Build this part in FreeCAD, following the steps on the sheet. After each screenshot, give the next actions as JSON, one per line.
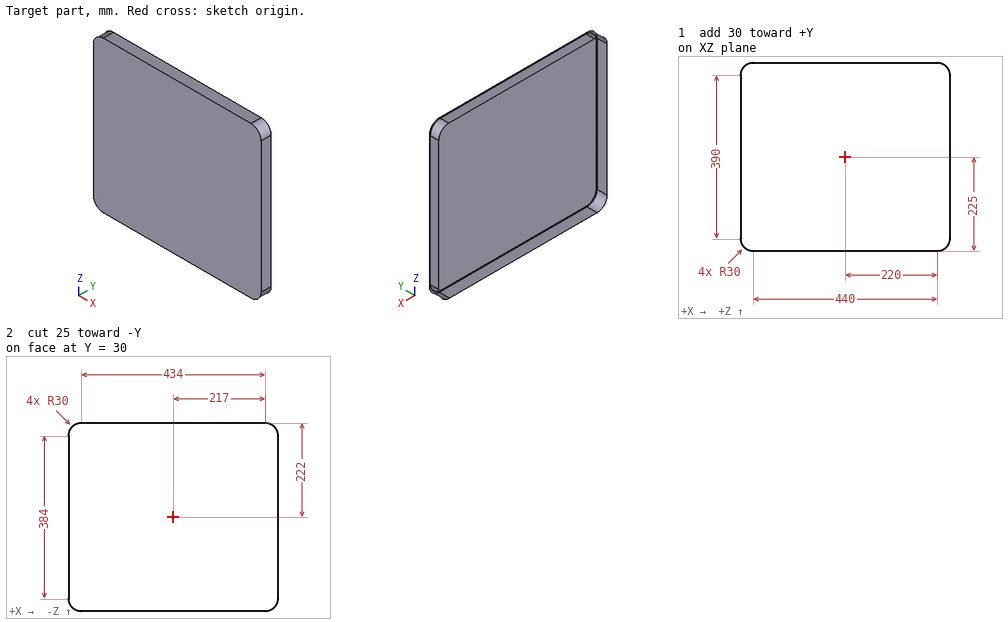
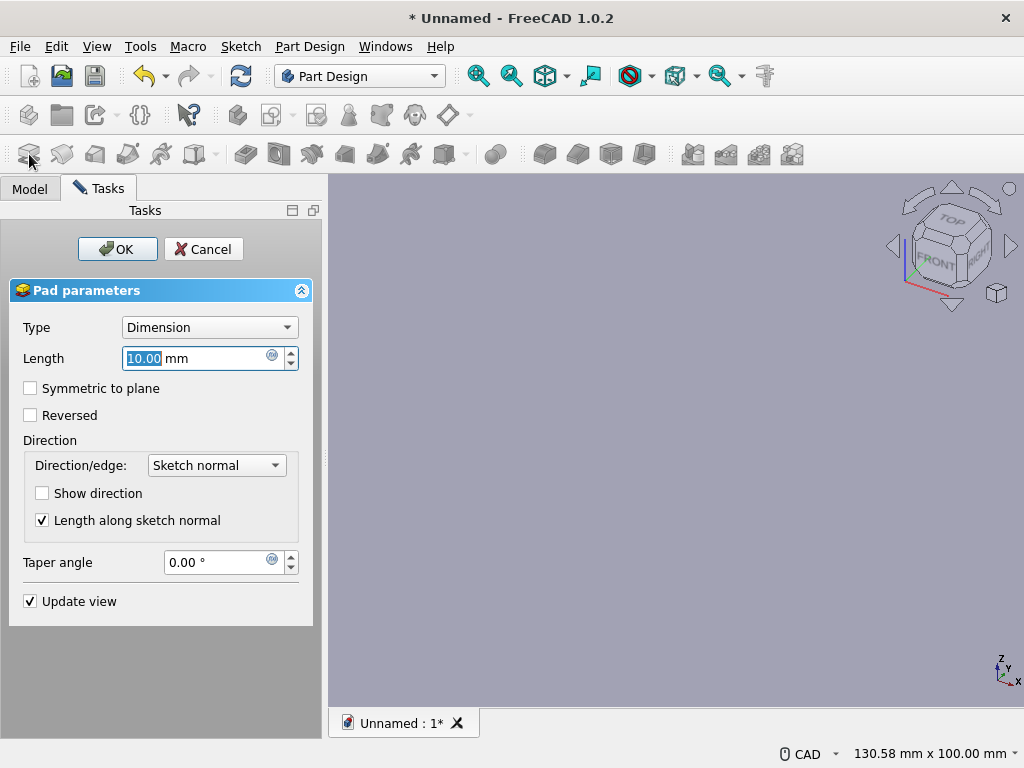
{"action": "type", "text": "30"}
{"action": "key", "text": "Tab"}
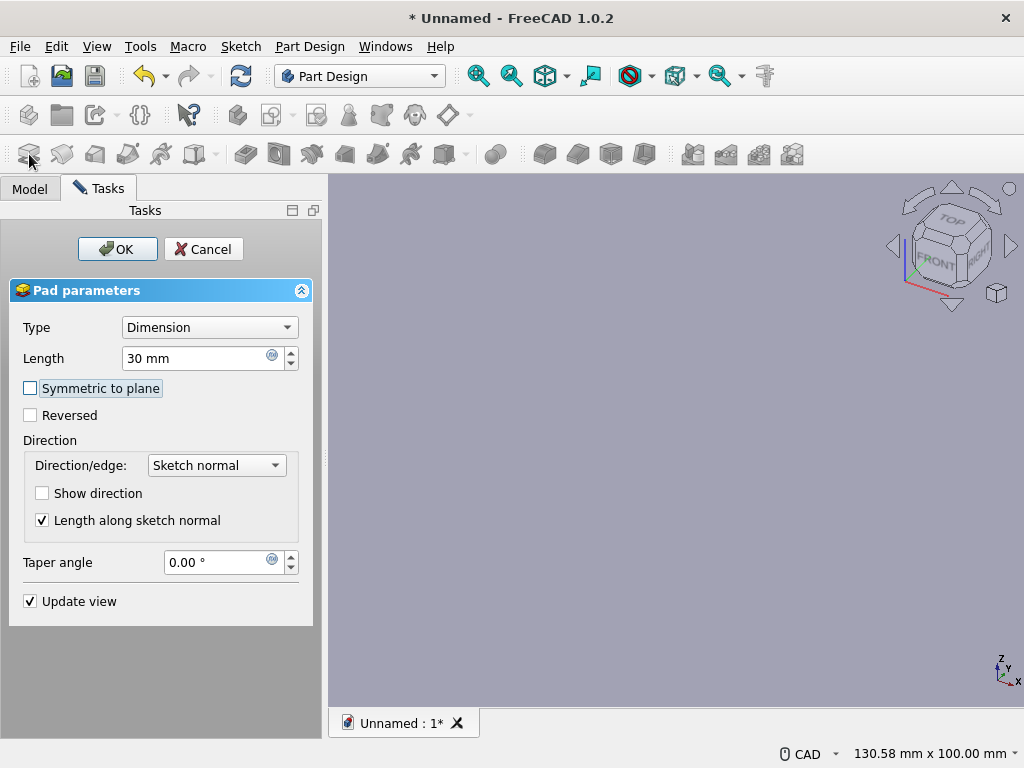
{"action": "left_click", "coordinate": [31, 415]}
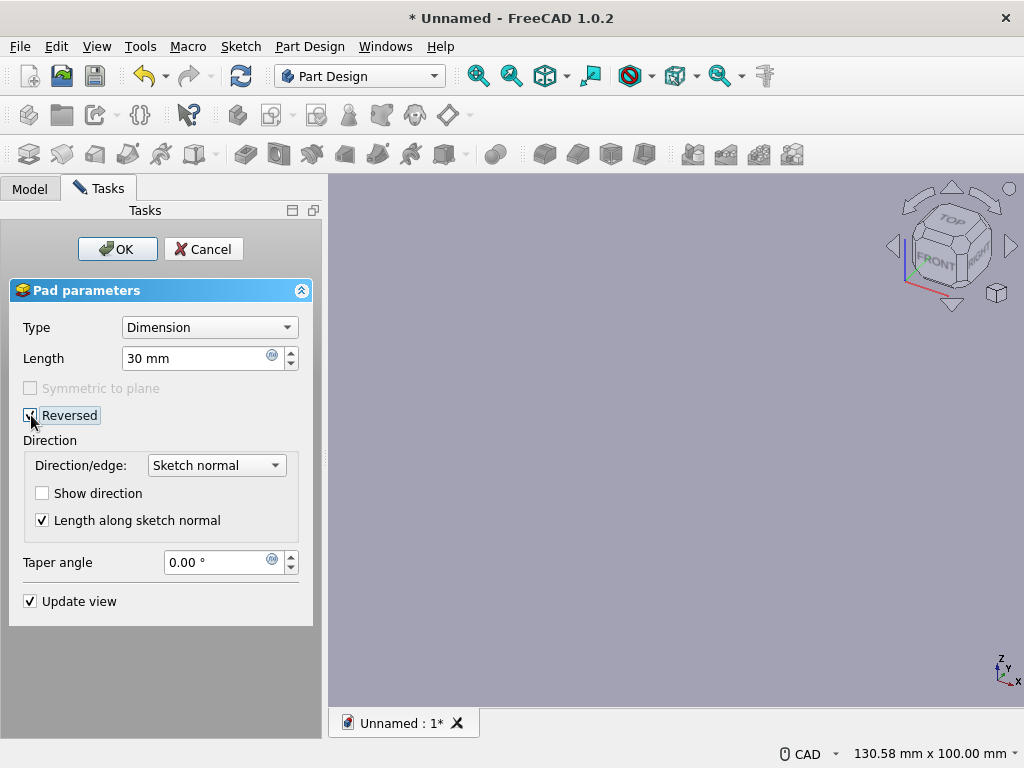
{"action": "left_click", "coordinate": [118, 249]}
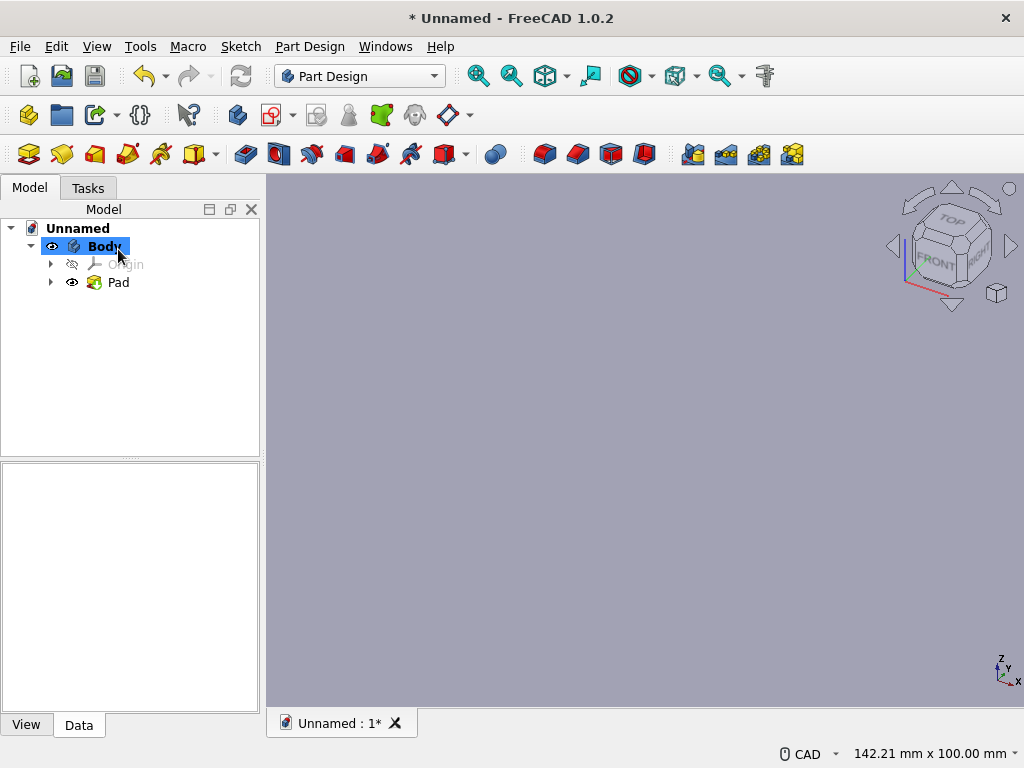
{"action": "left_click", "coordinate": [479, 76]}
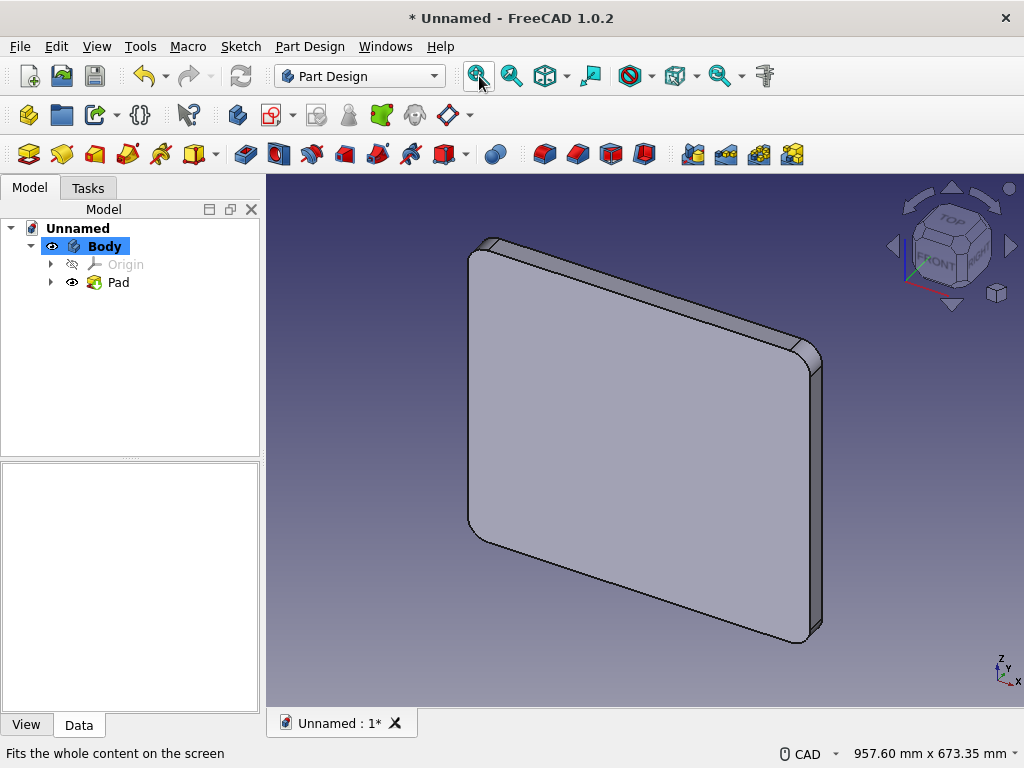
{"action": "key", "text": "4"}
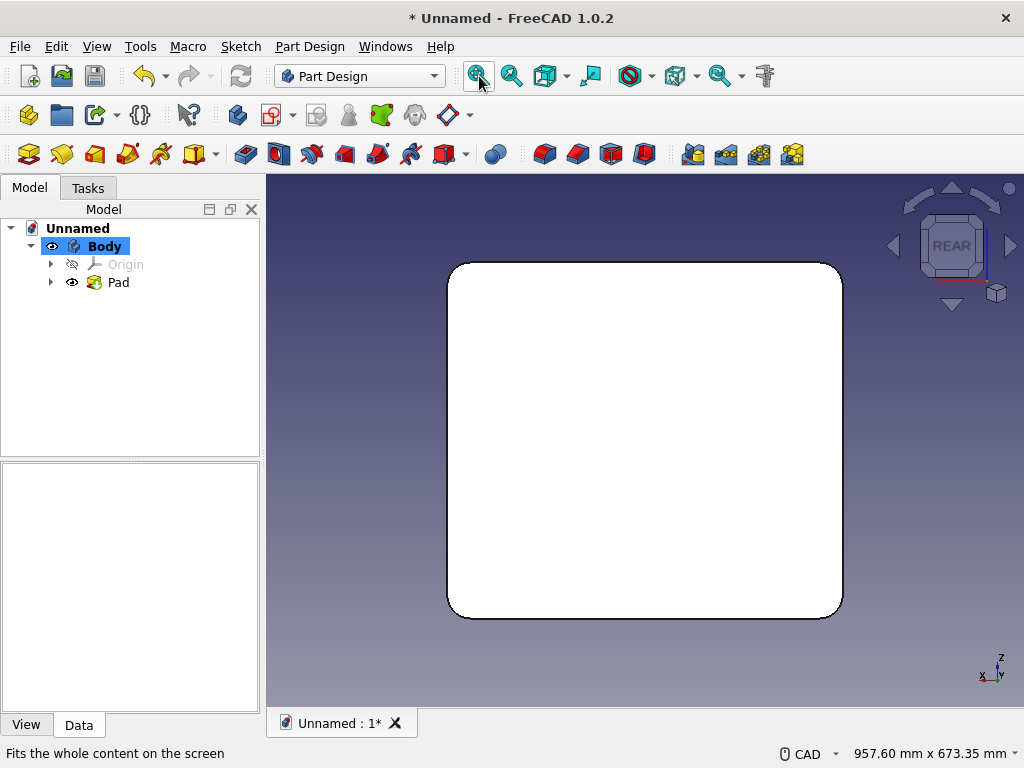
{"action": "left_click", "coordinate": [645, 439]}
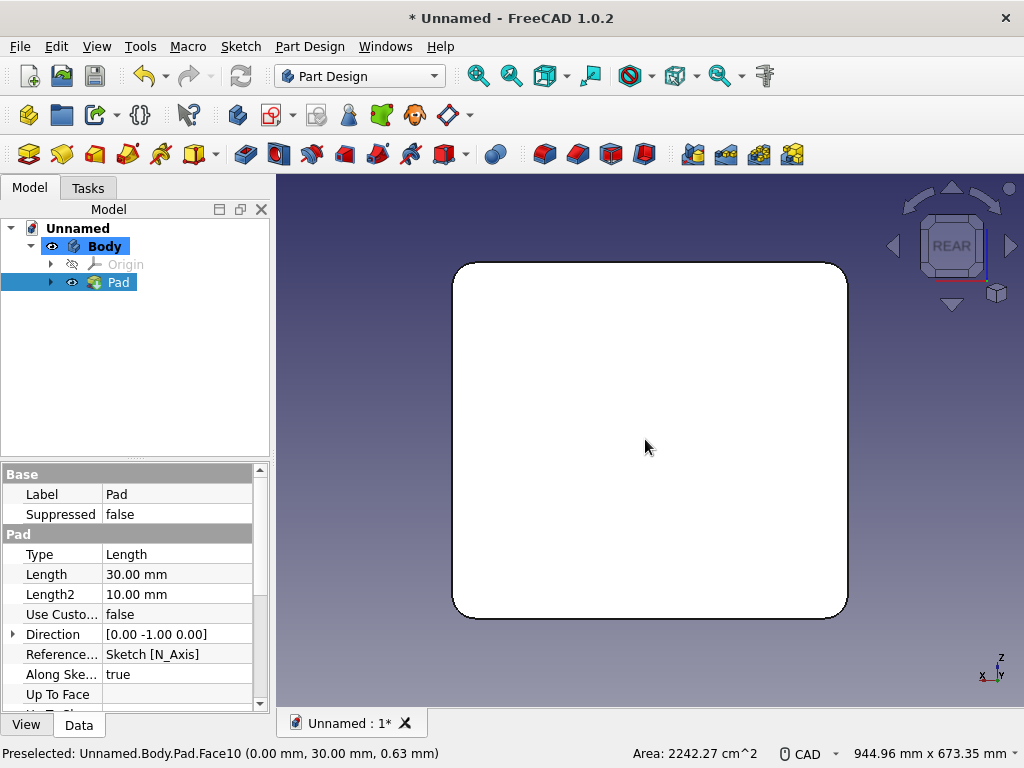
{"action": "left_click", "coordinate": [270, 116]}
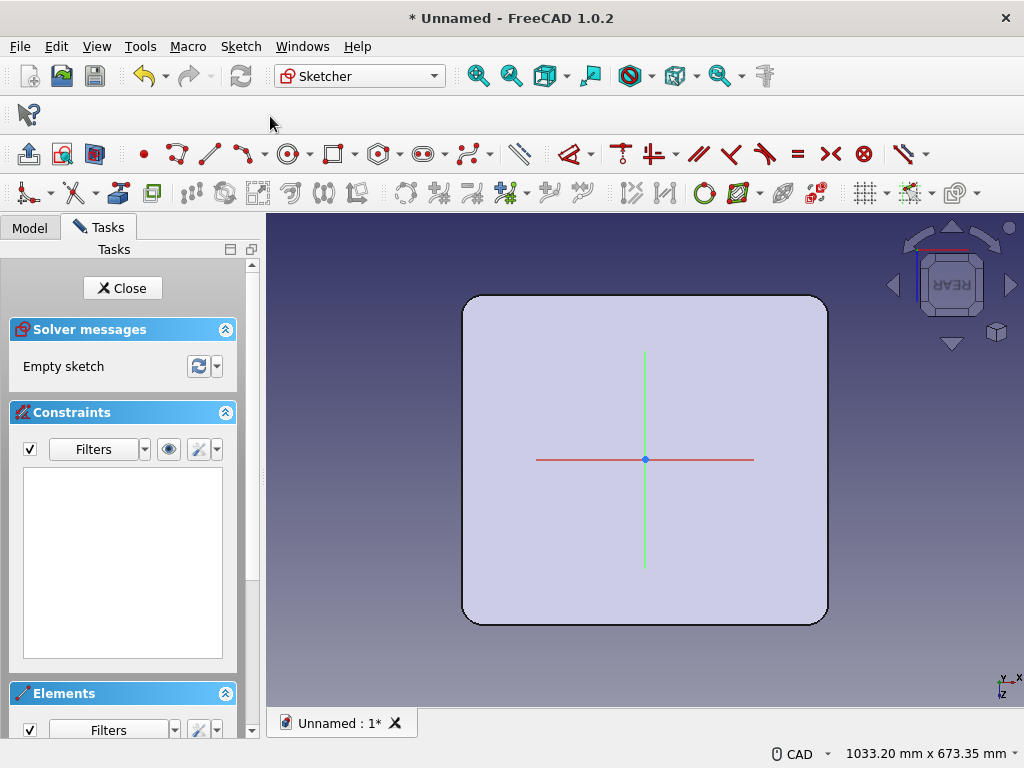
{"action": "left_click", "coordinate": [210, 154]}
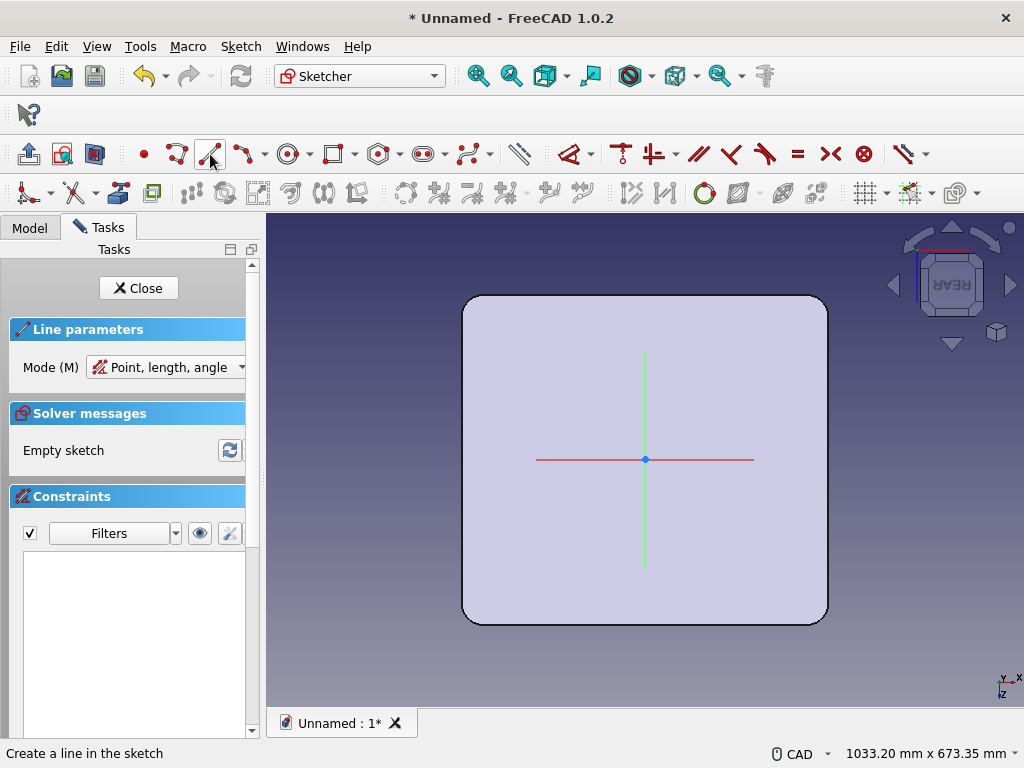
{"action": "left_click", "coordinate": [804, 297]}
{"action": "left_click", "coordinate": [486, 297]}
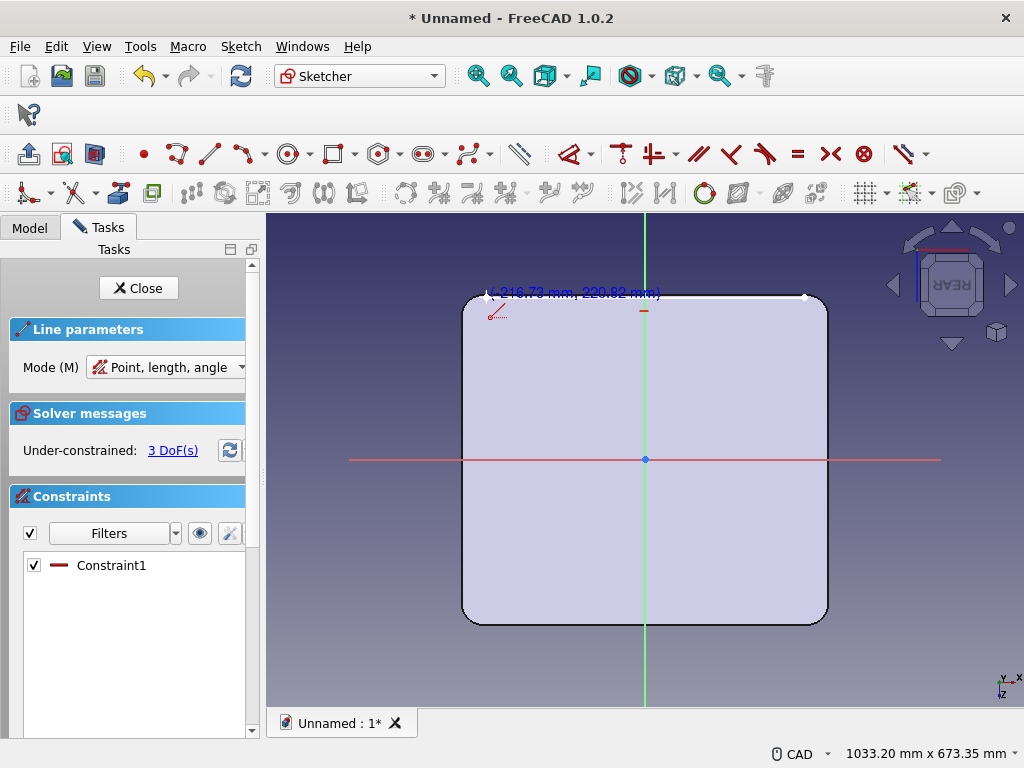
{"action": "left_click", "coordinate": [464, 319]}
{"action": "left_click", "coordinate": [464, 601]}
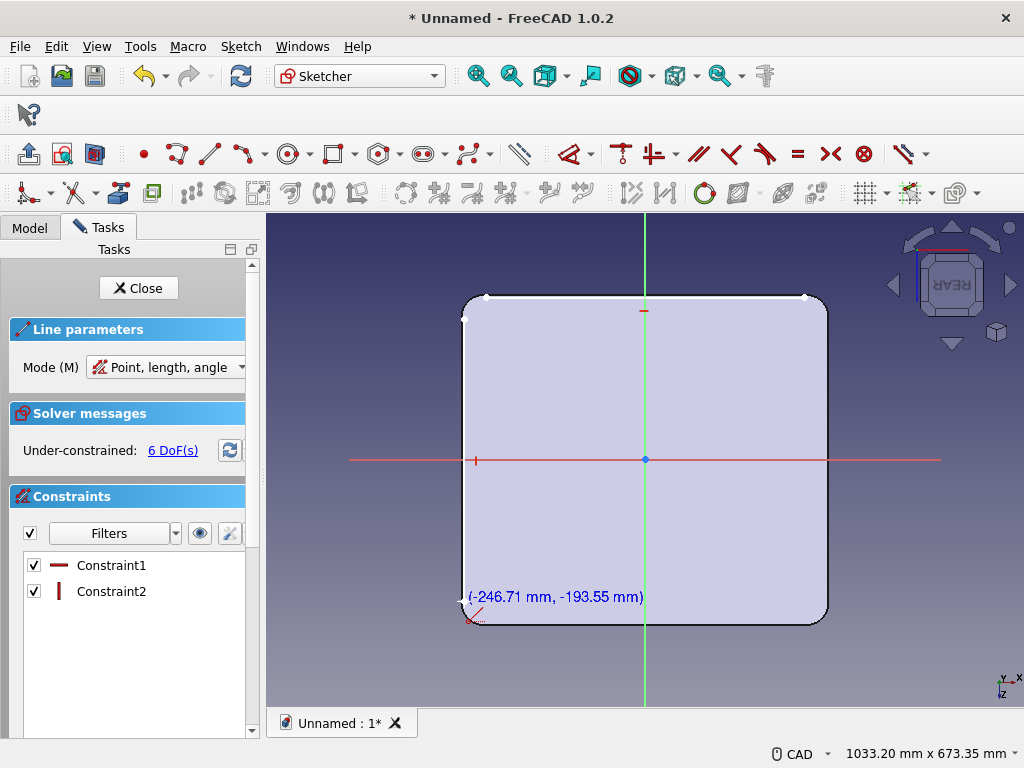
{"action": "left_click", "coordinate": [486, 623]}
{"action": "left_click", "coordinate": [804, 623]}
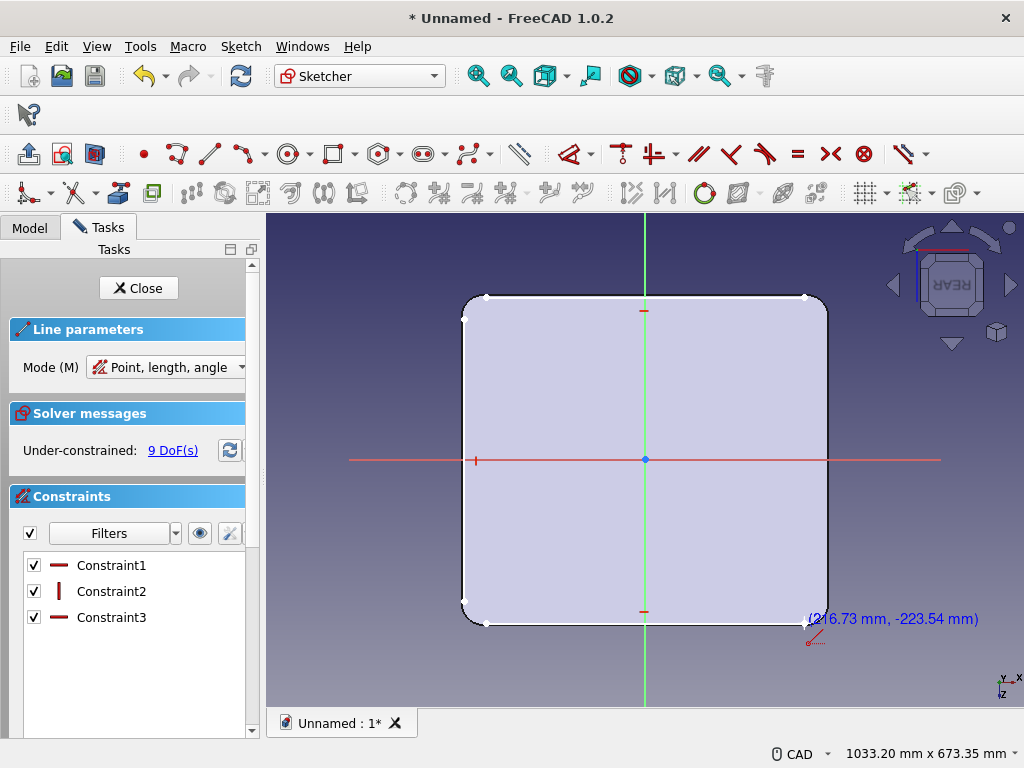
{"action": "left_click", "coordinate": [826, 601]}
{"action": "left_click", "coordinate": [826, 319]}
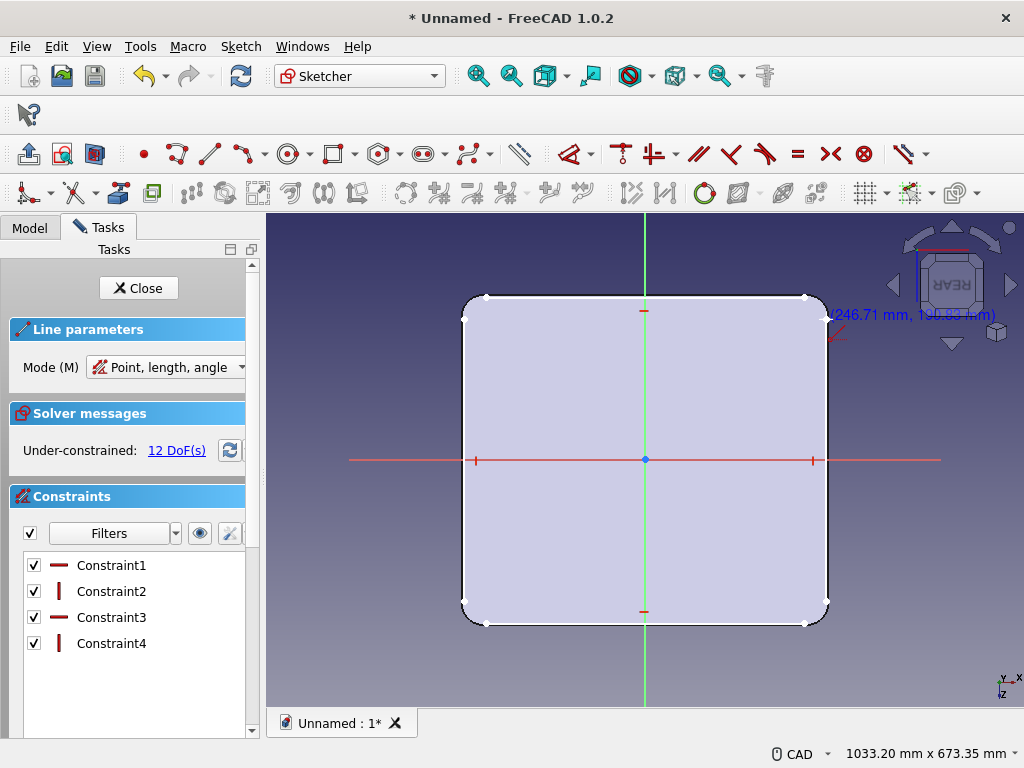
{"action": "left_click", "coordinate": [242, 154]}